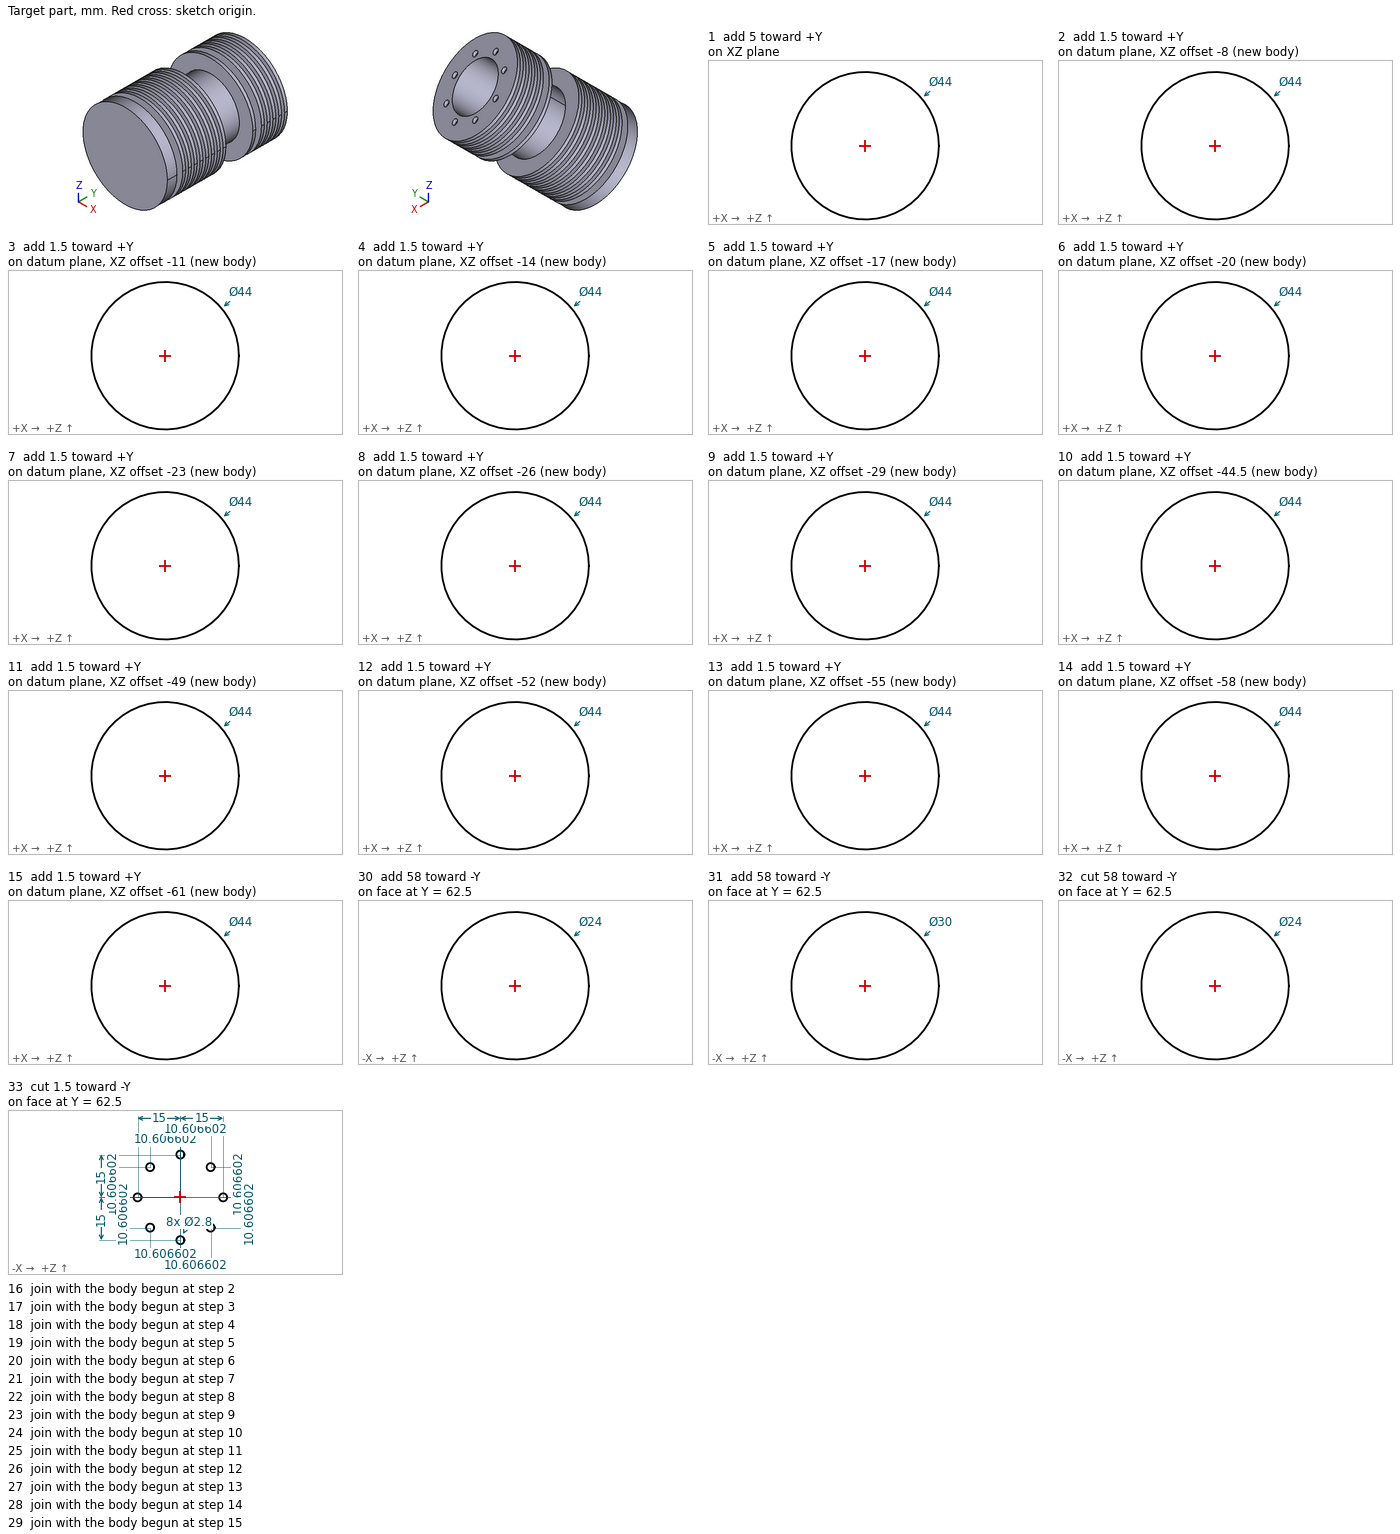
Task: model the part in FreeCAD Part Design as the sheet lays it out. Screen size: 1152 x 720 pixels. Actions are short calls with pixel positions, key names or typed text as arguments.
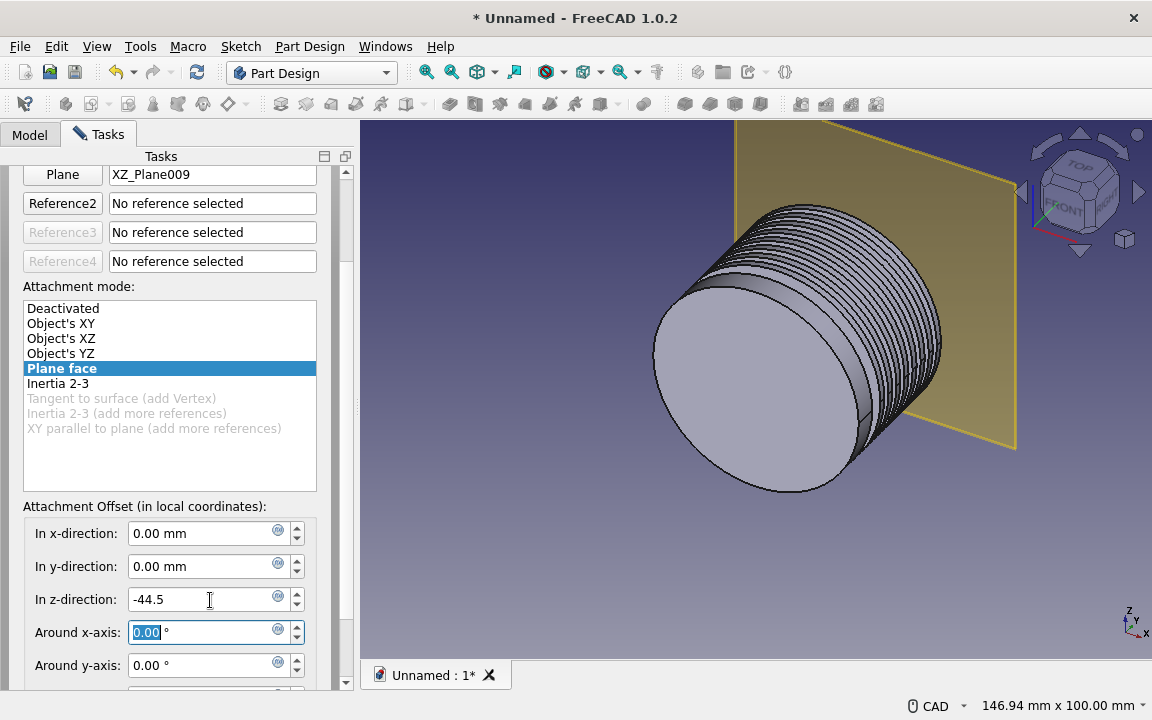
scroll(346, 428, up, 3)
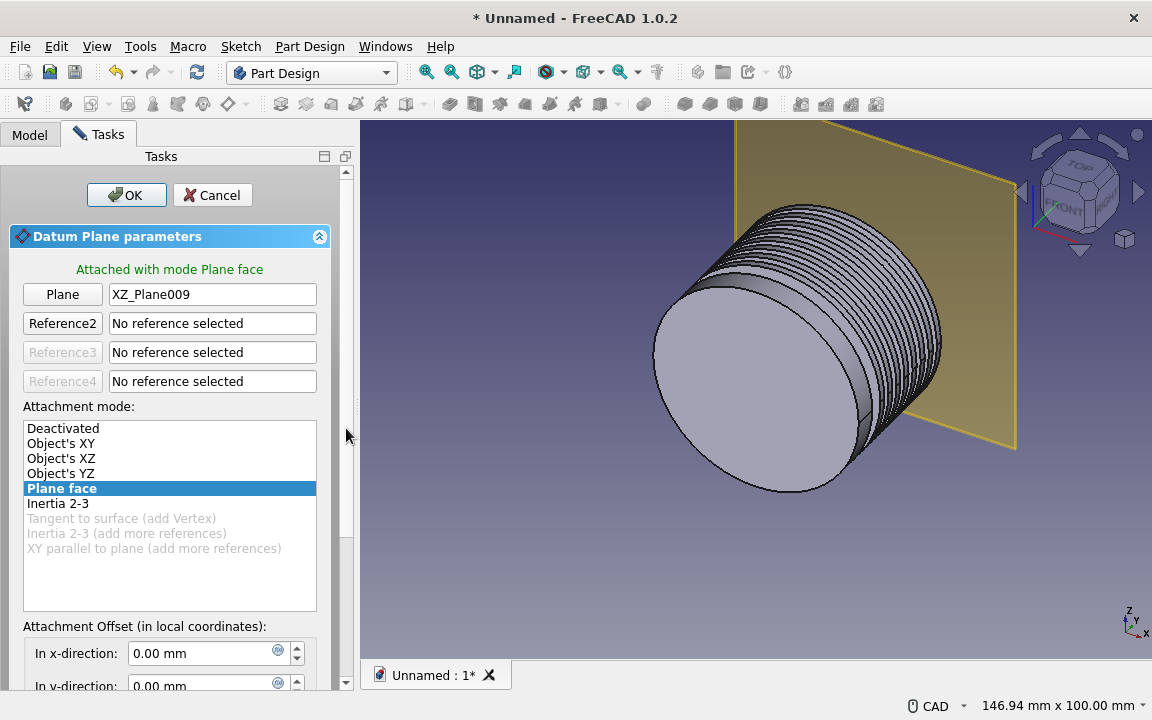
click(127, 195)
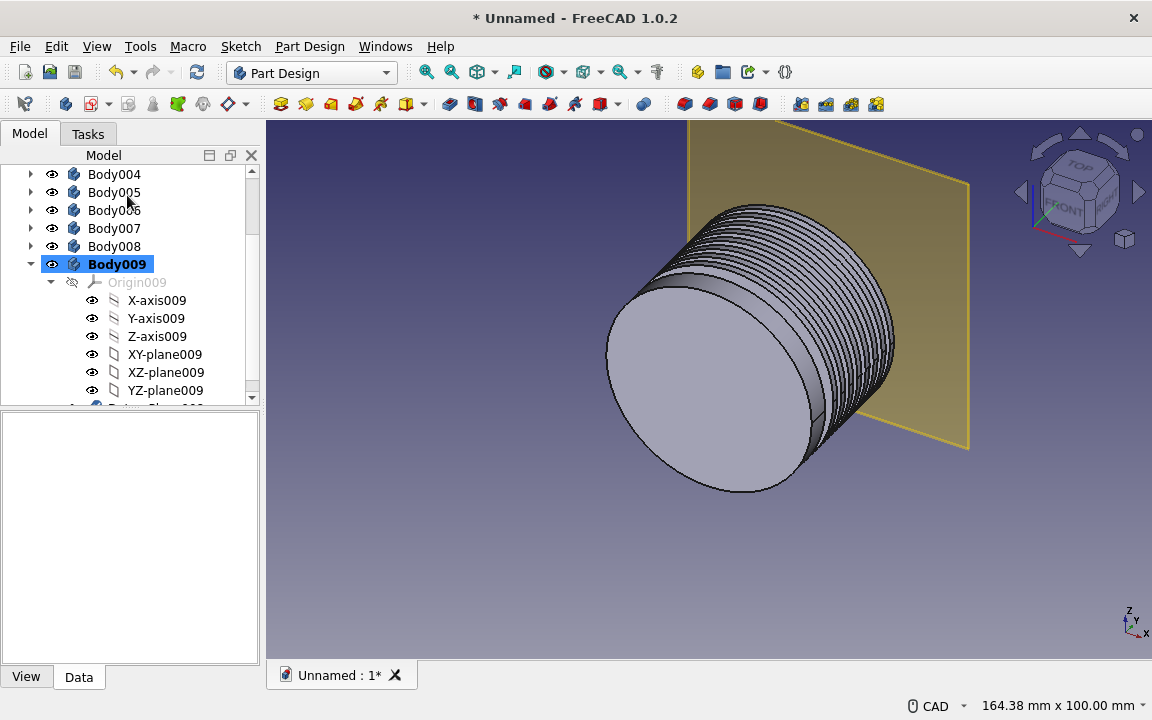
scroll(121, 278, down, 3)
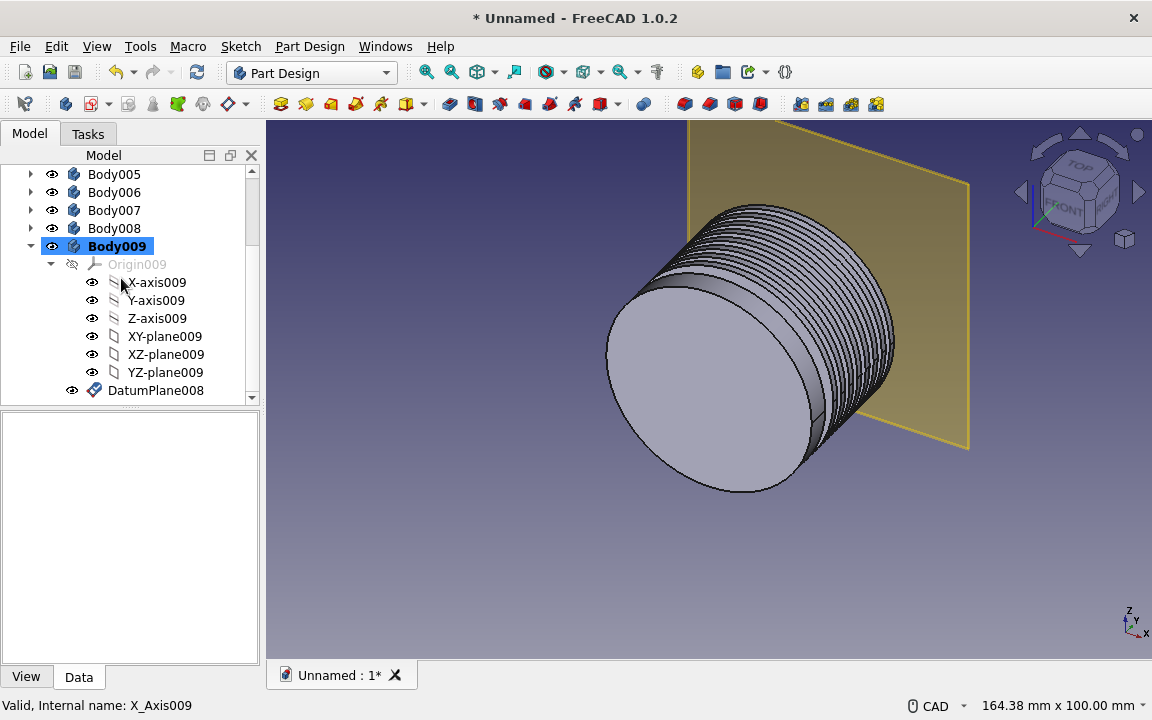
click(117, 390)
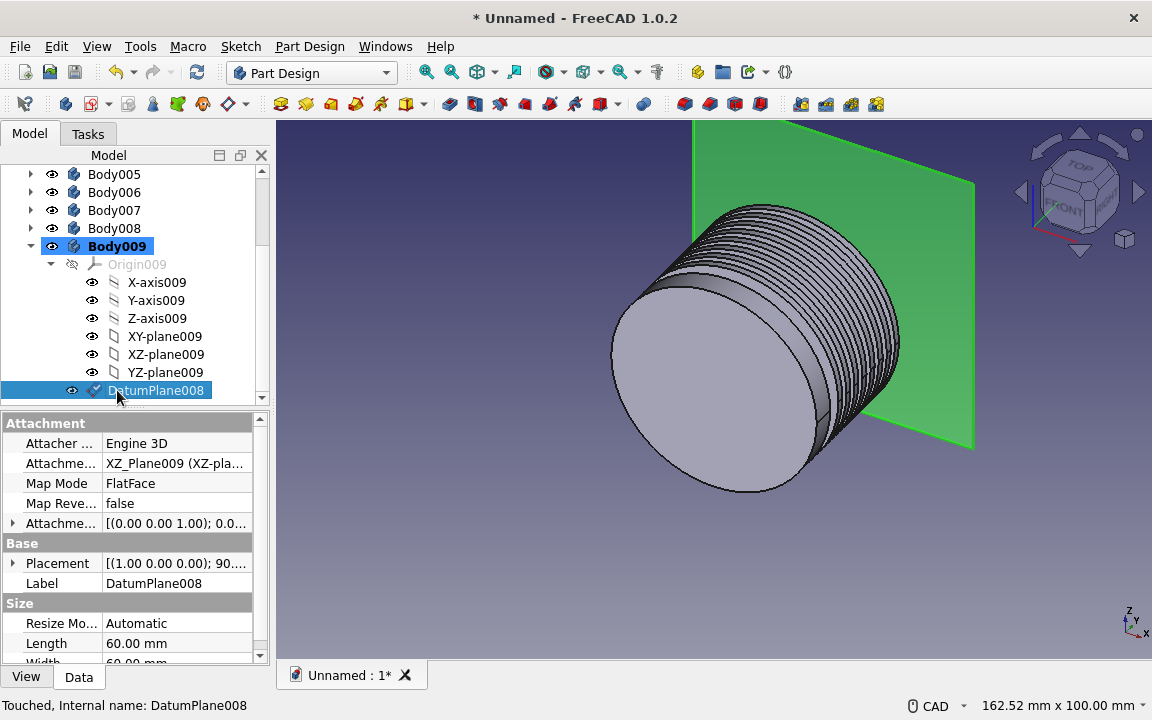
click(90, 104)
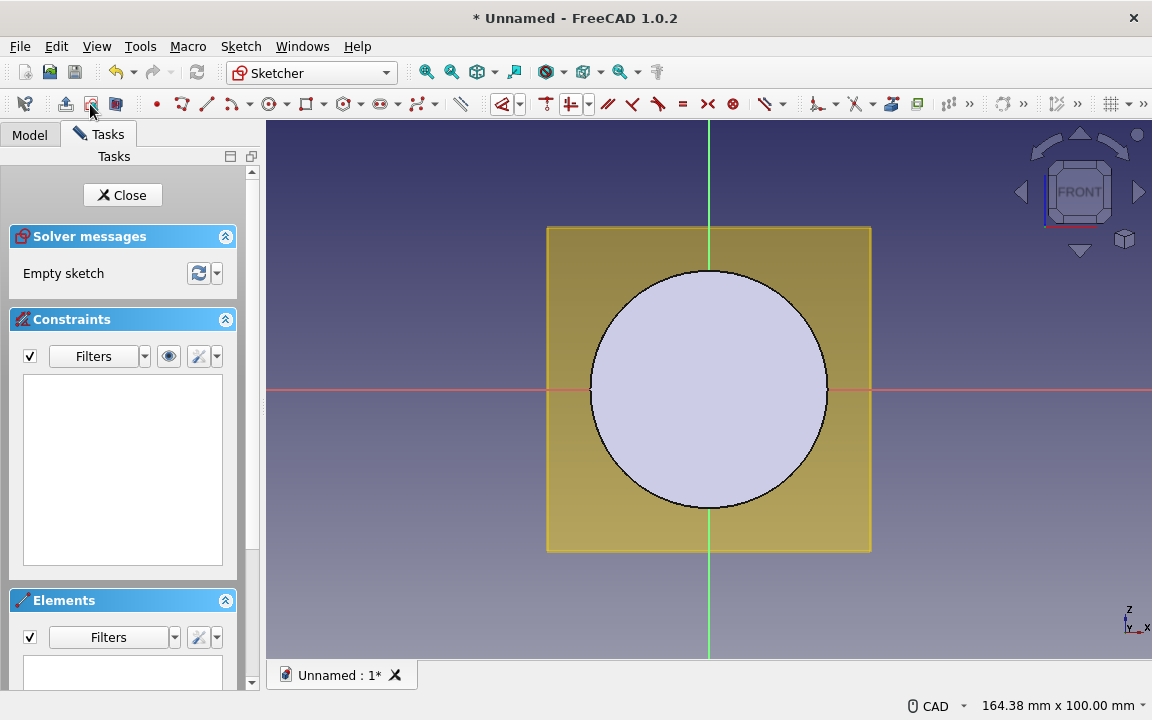
scroll(848, 390, up, 2)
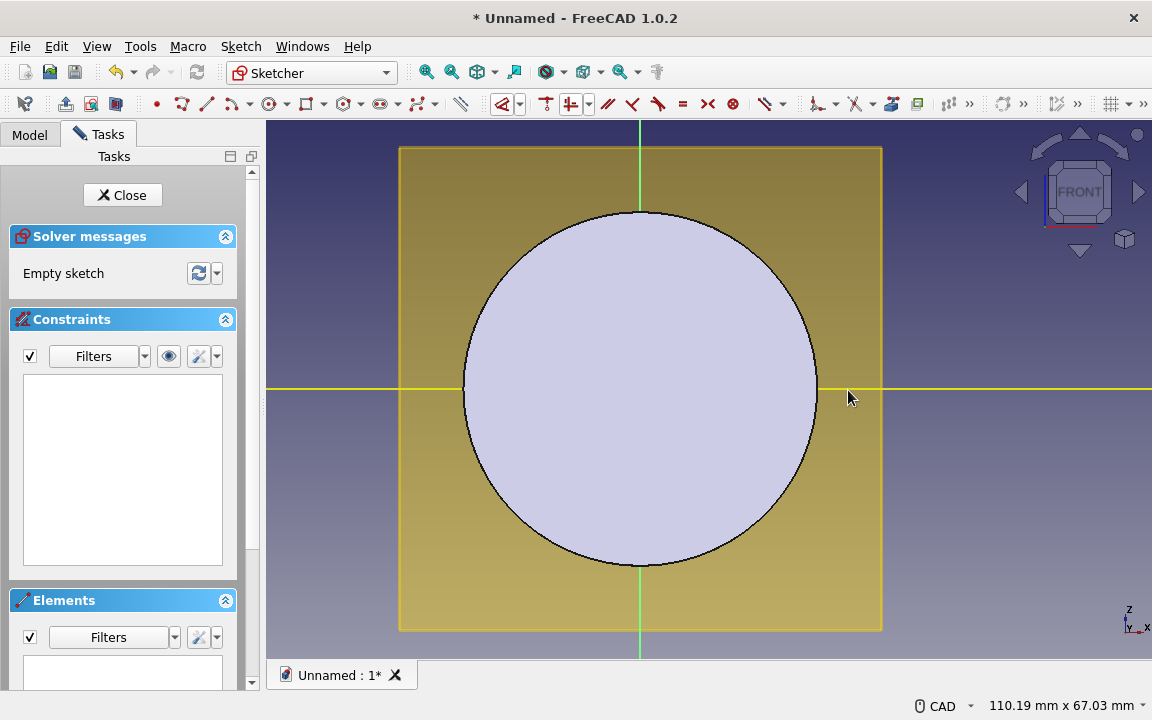
key(g)
key(c)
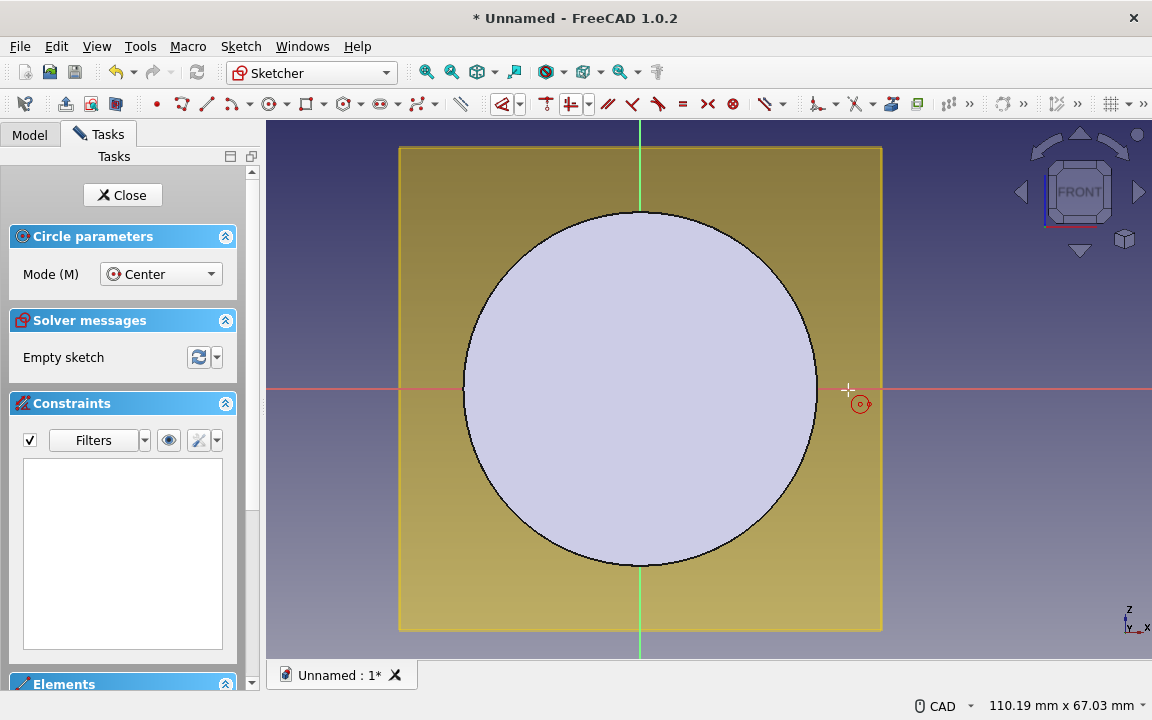
click(640, 389)
click(765, 264)
key(Escape)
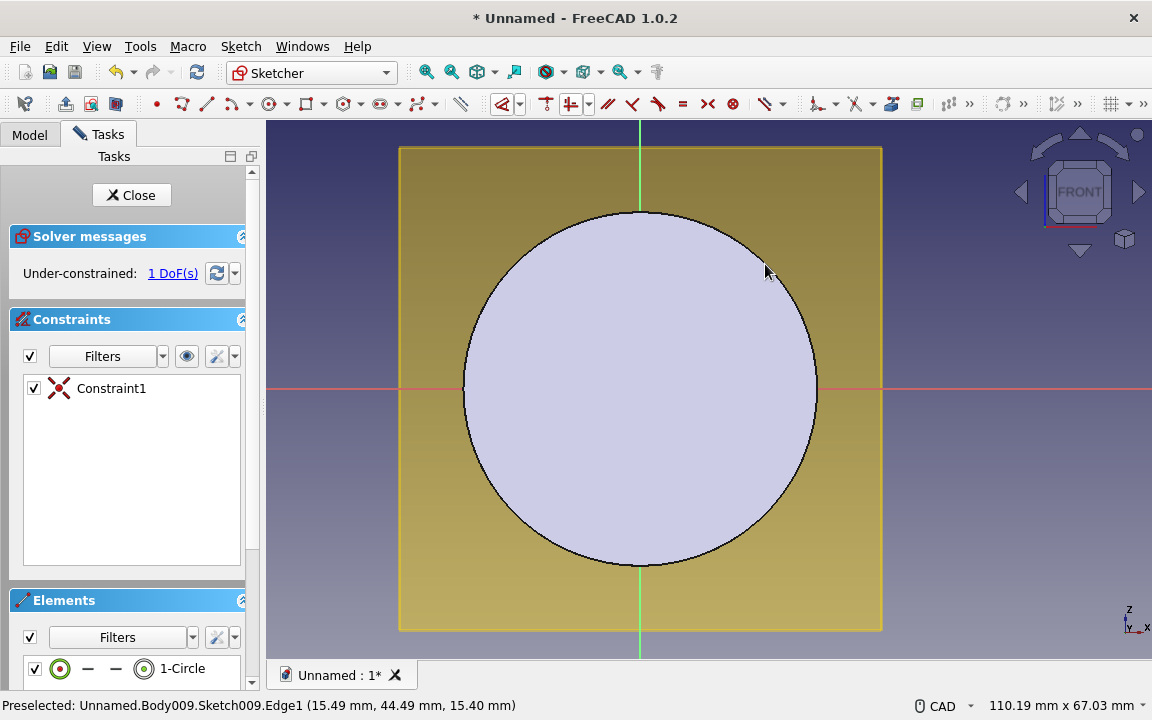
click(764, 264)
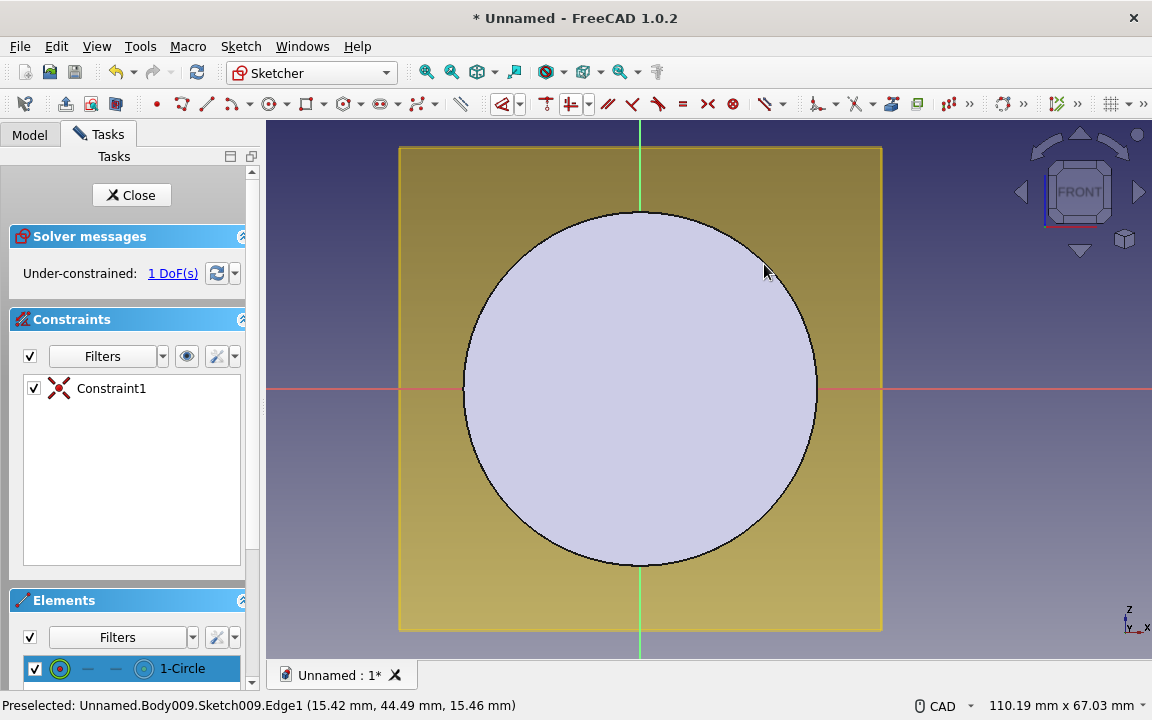
key(k)
key(o)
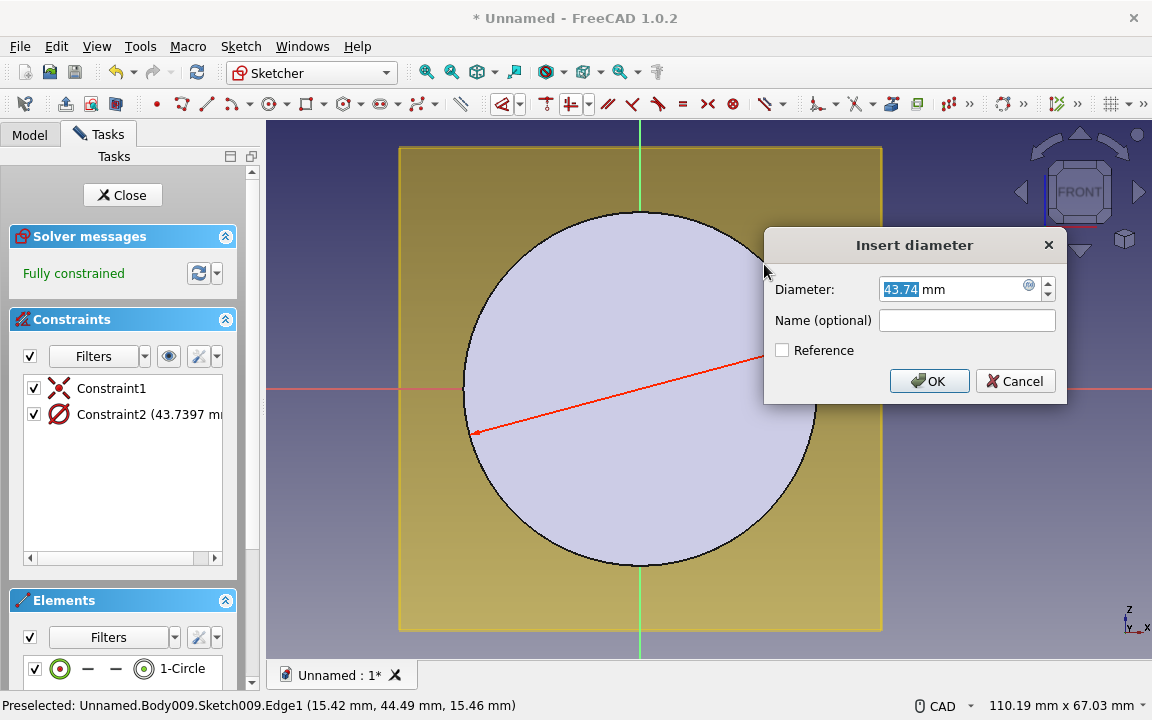
text(44)
key(Return)